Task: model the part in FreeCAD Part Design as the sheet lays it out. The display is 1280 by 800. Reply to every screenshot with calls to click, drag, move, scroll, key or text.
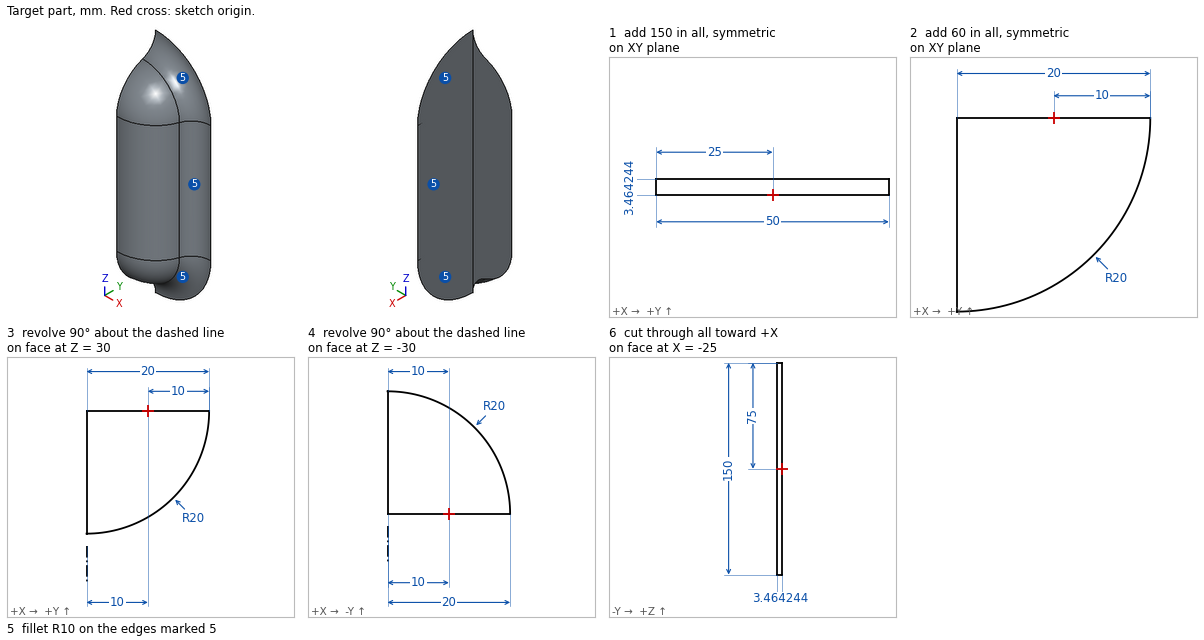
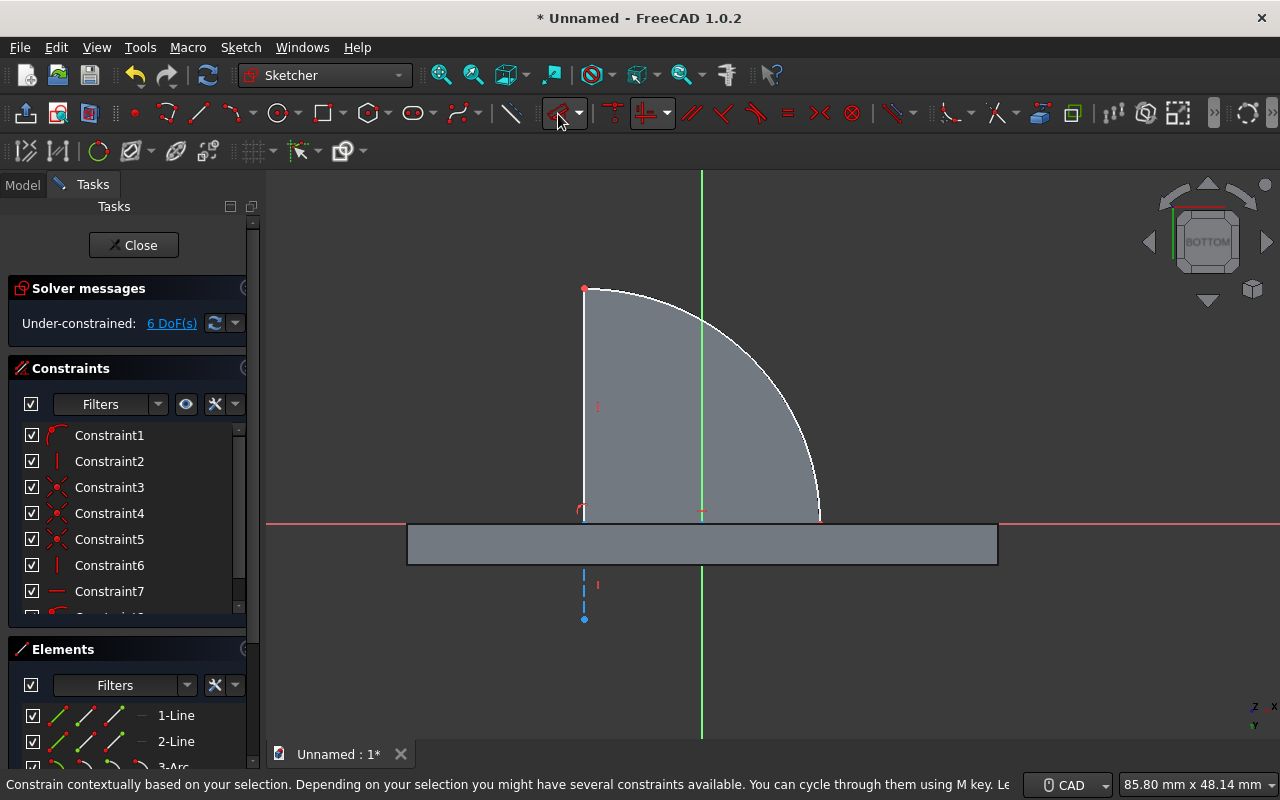
click(794, 417)
click(822, 402)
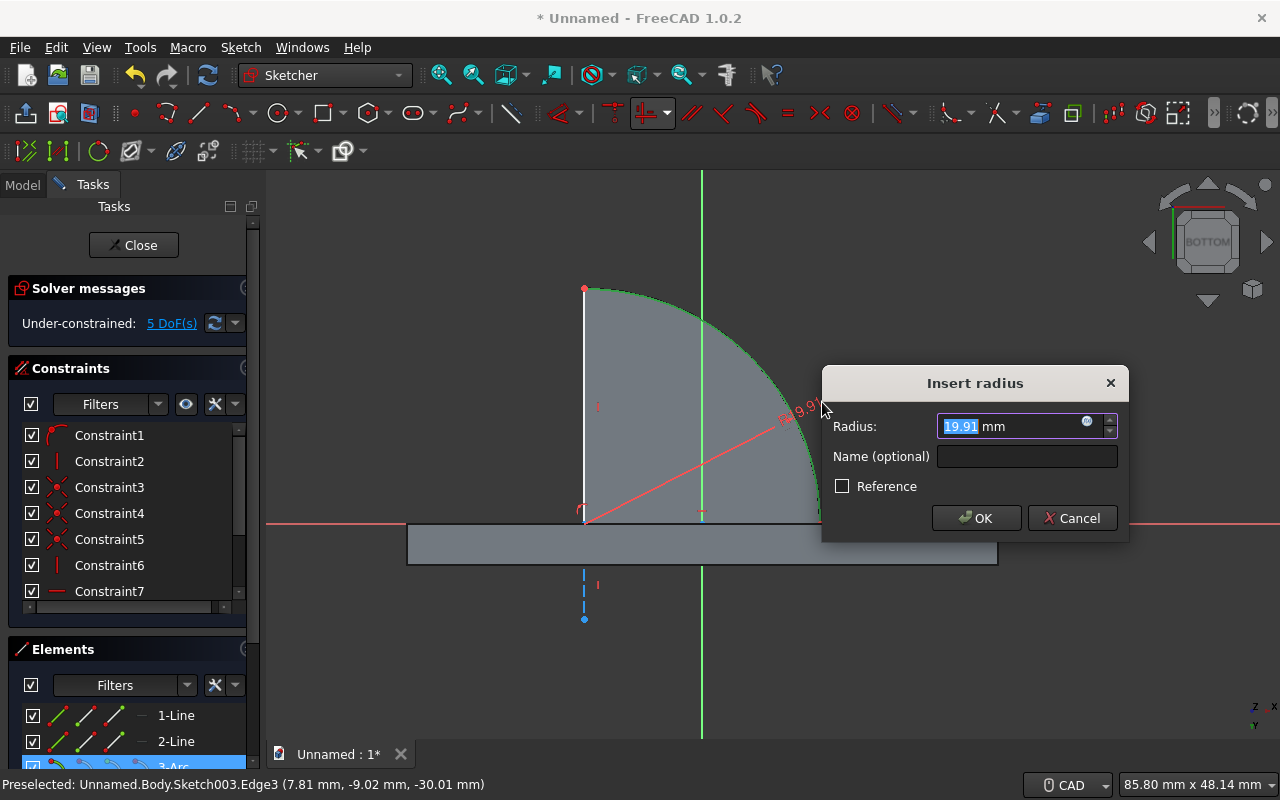
text(20)
key(Return)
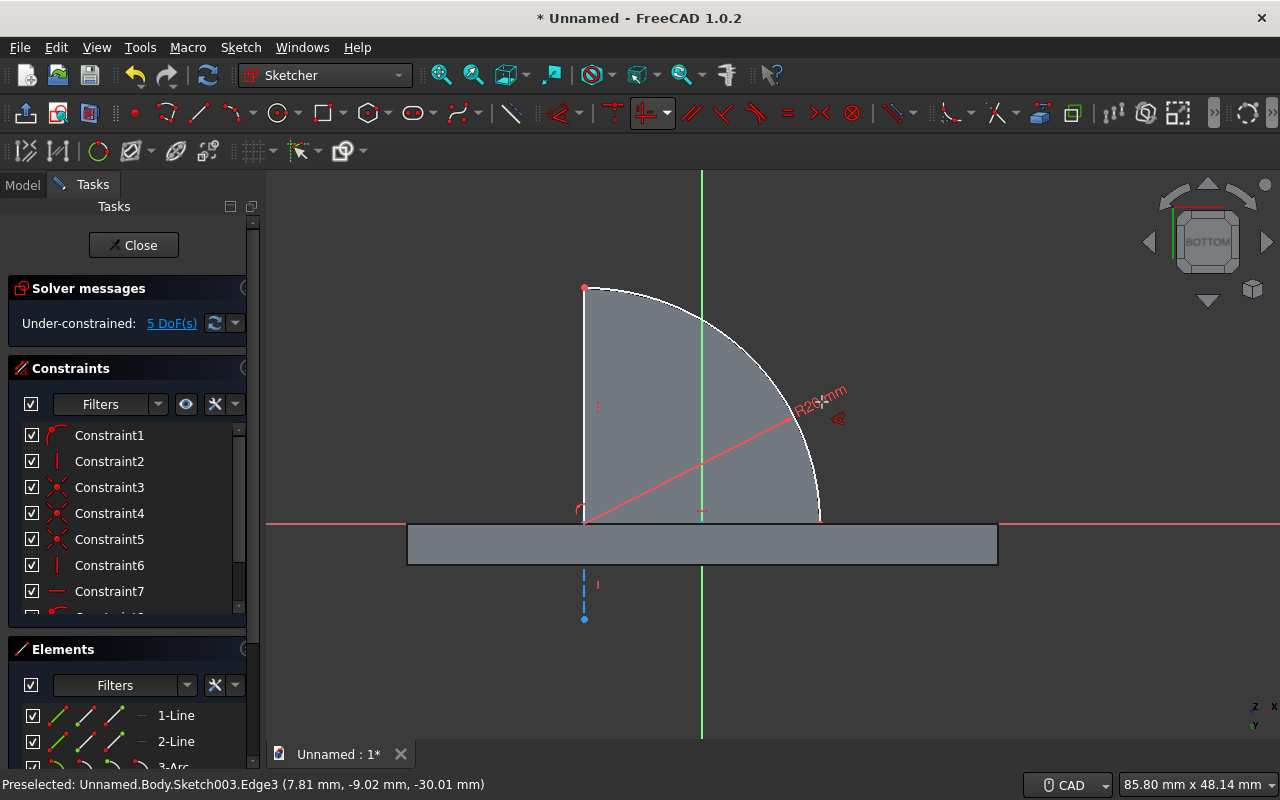
click(655, 524)
click(648, 558)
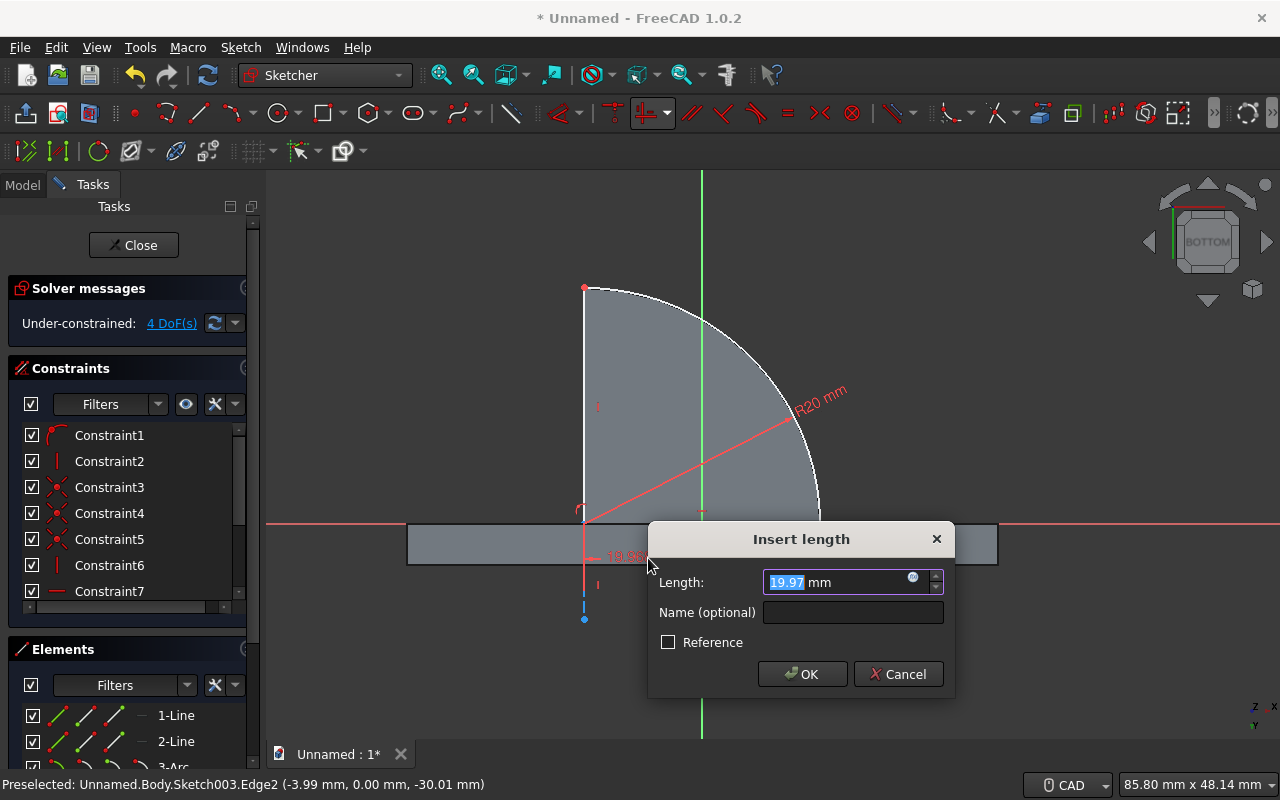
text(20)
key(Return)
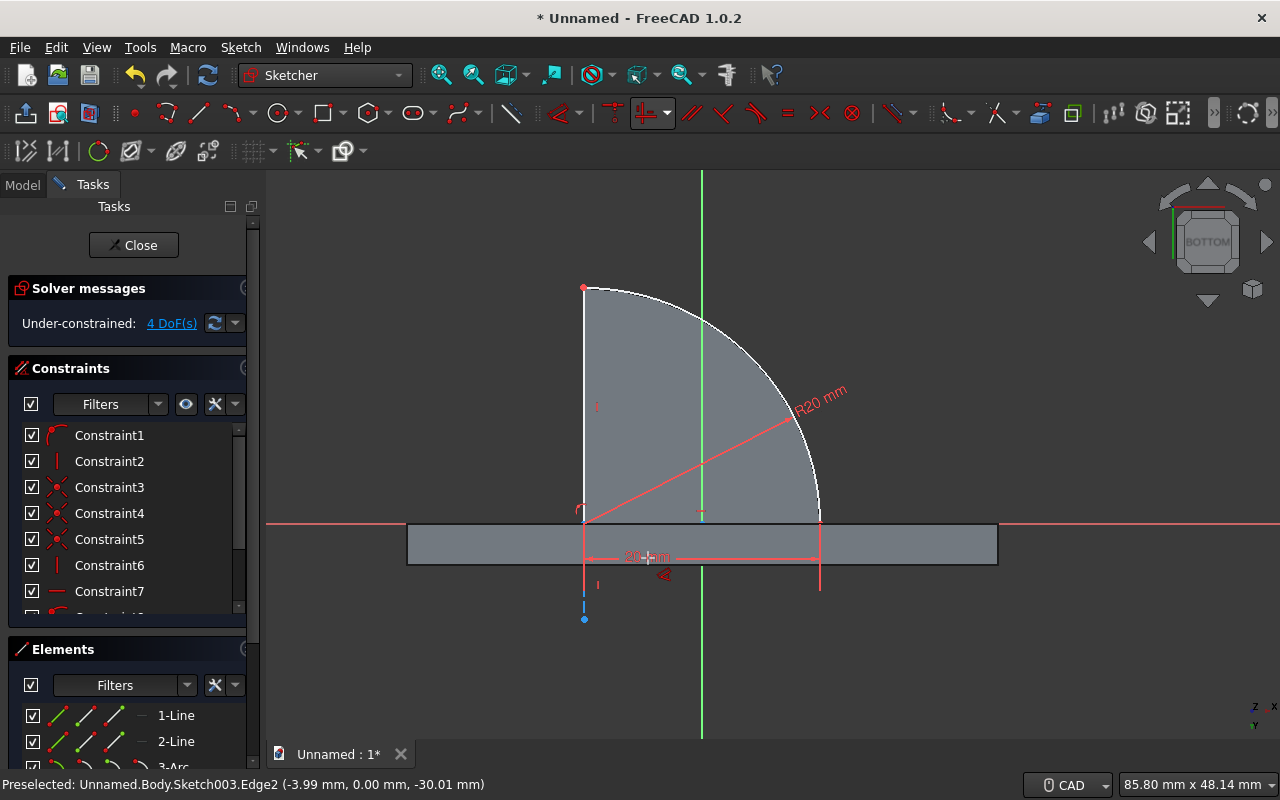
click(584, 288)
click(643, 254)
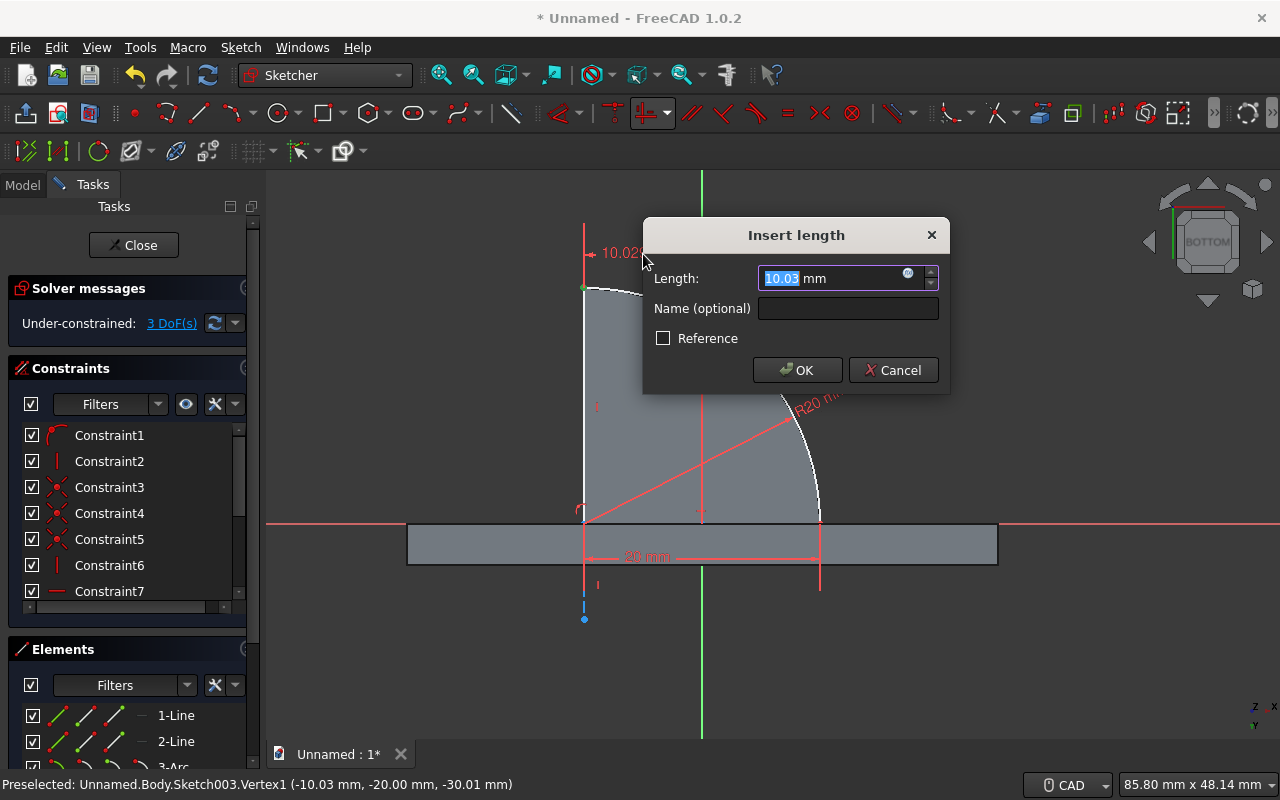
text(10)
key(Return)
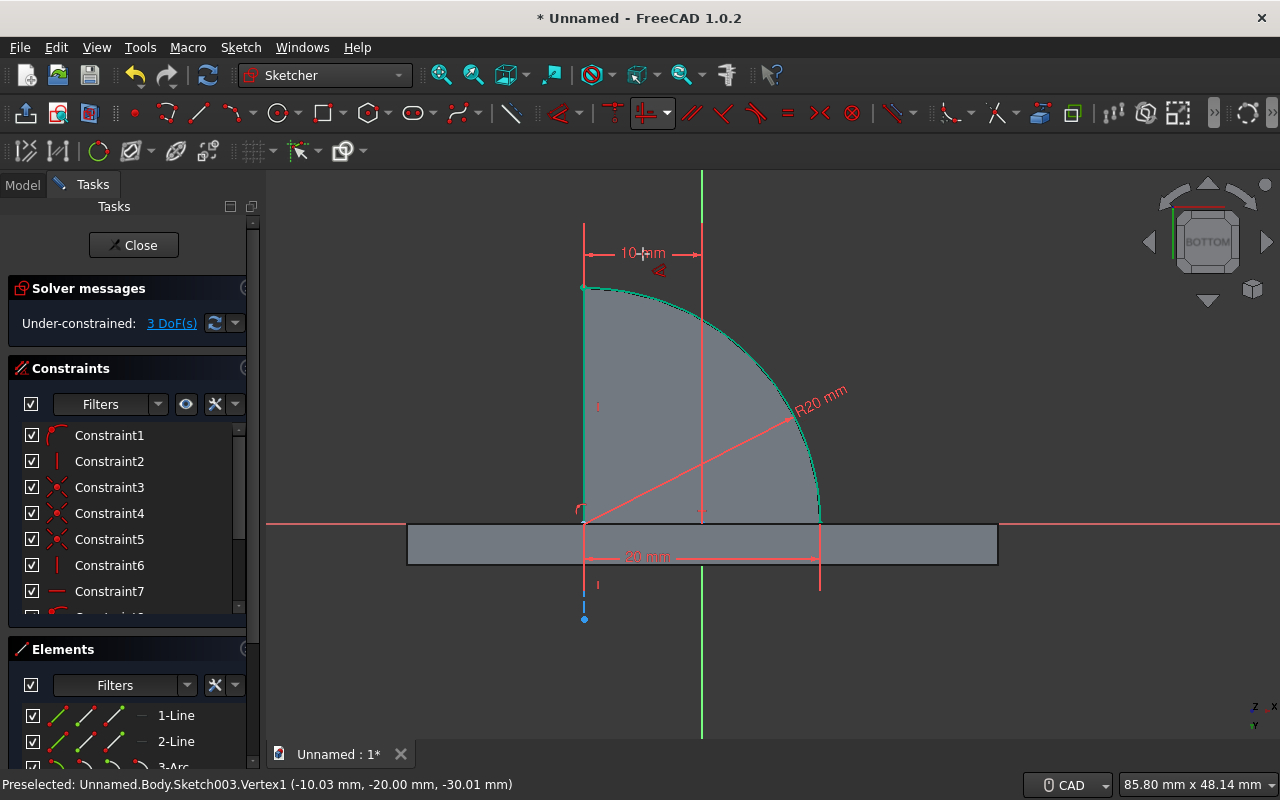
click(584, 549)
click(643, 583)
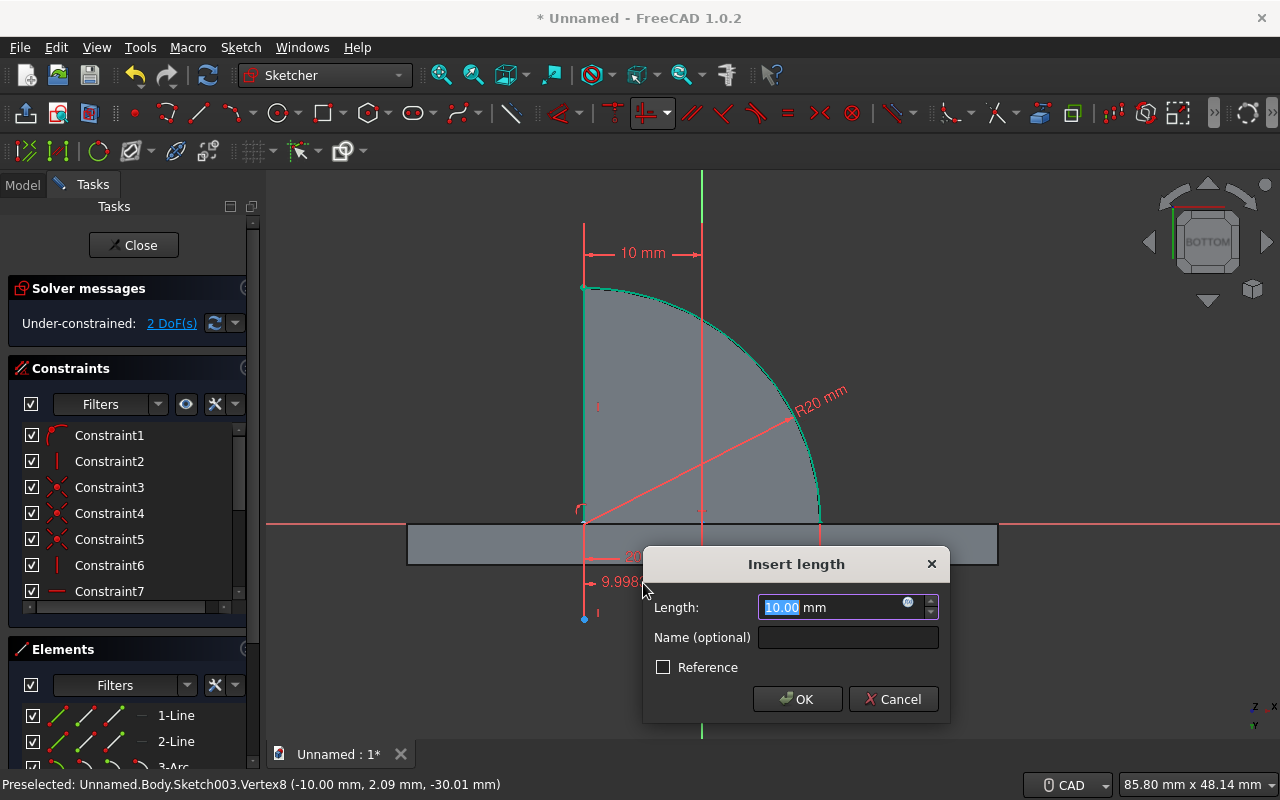
text(10)
key(Return)
key(Escape)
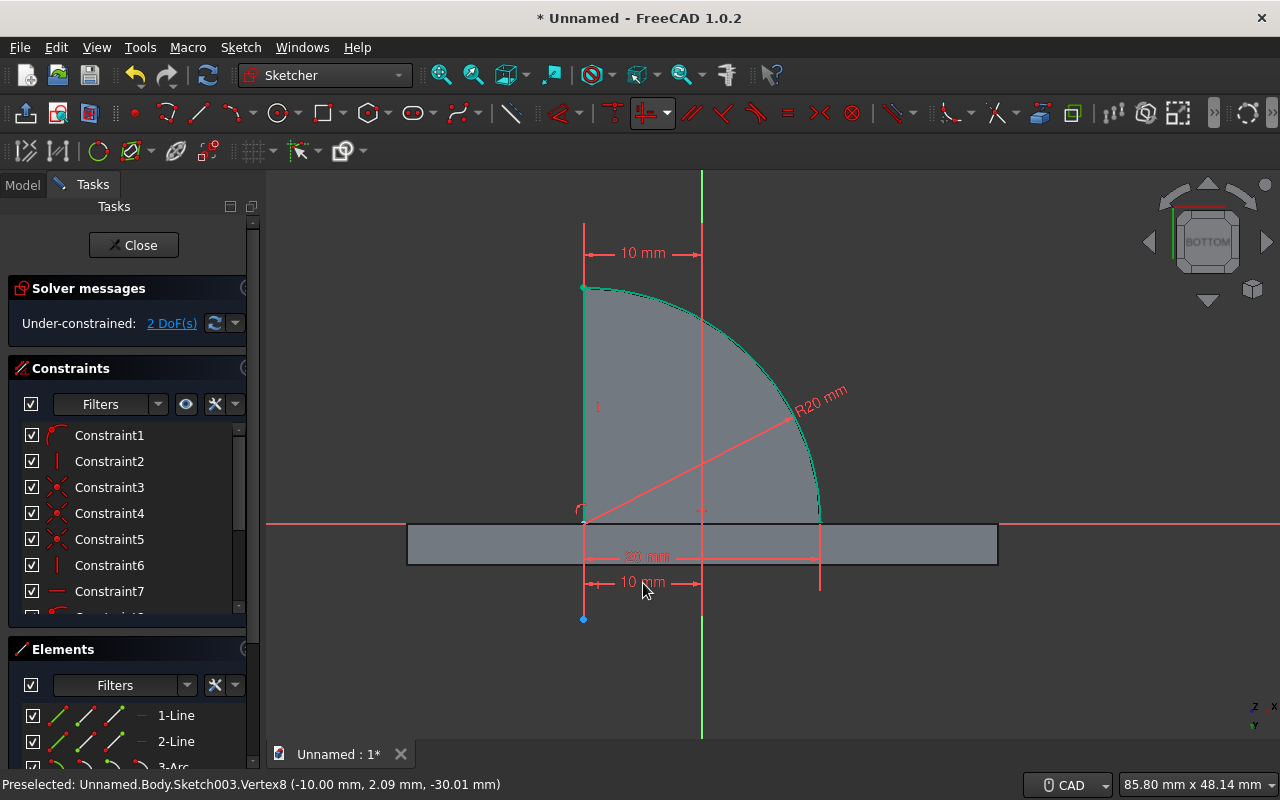
click(134, 245)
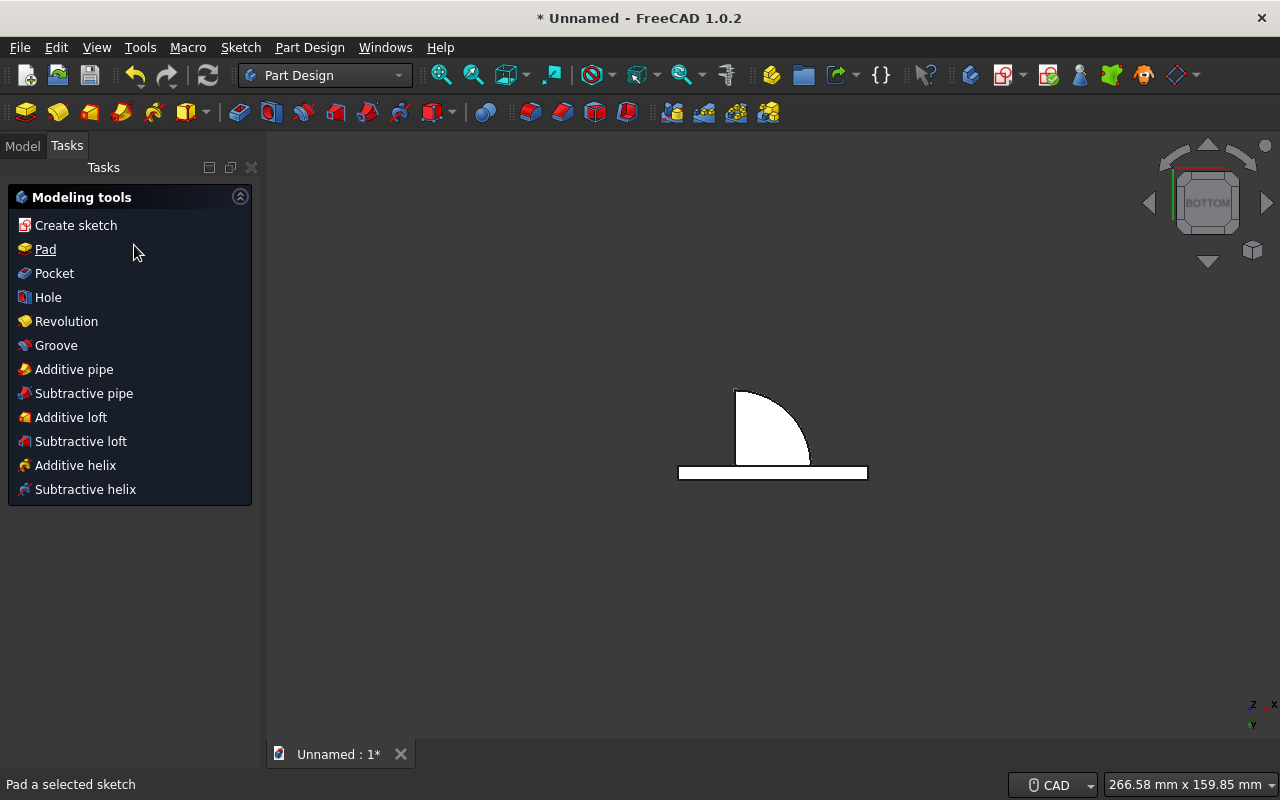
click(58, 112)